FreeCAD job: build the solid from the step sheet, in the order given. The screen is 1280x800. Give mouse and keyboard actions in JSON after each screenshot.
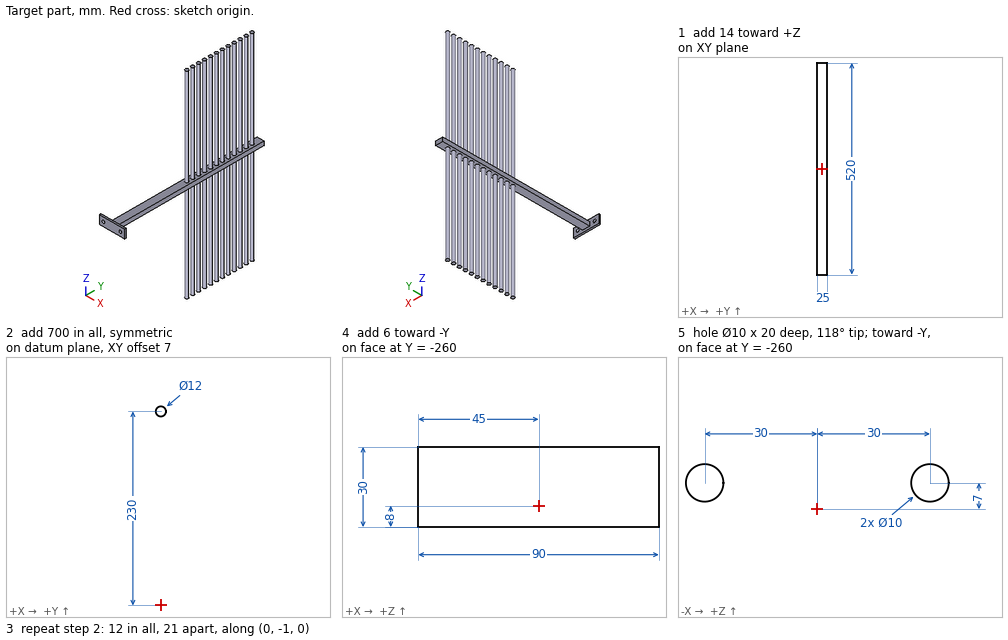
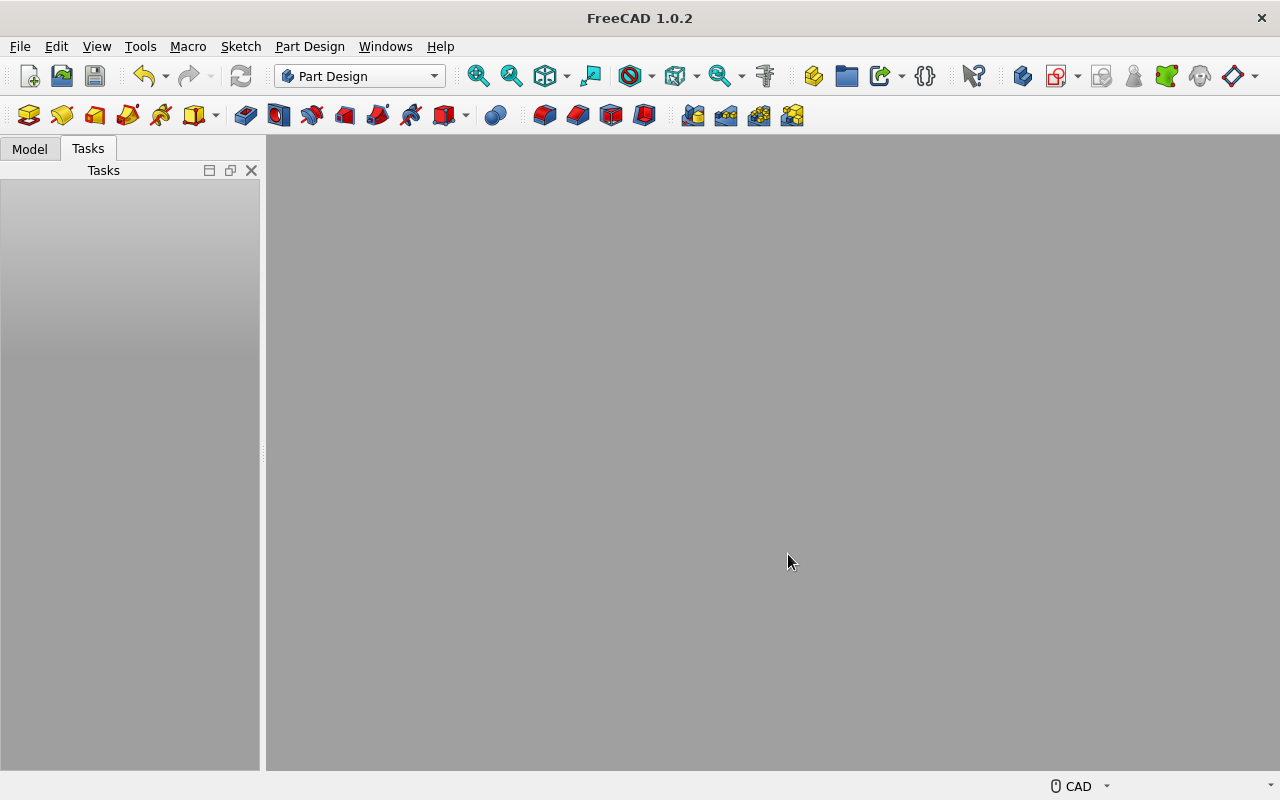
{"action": "left_click", "coordinate": [29, 76]}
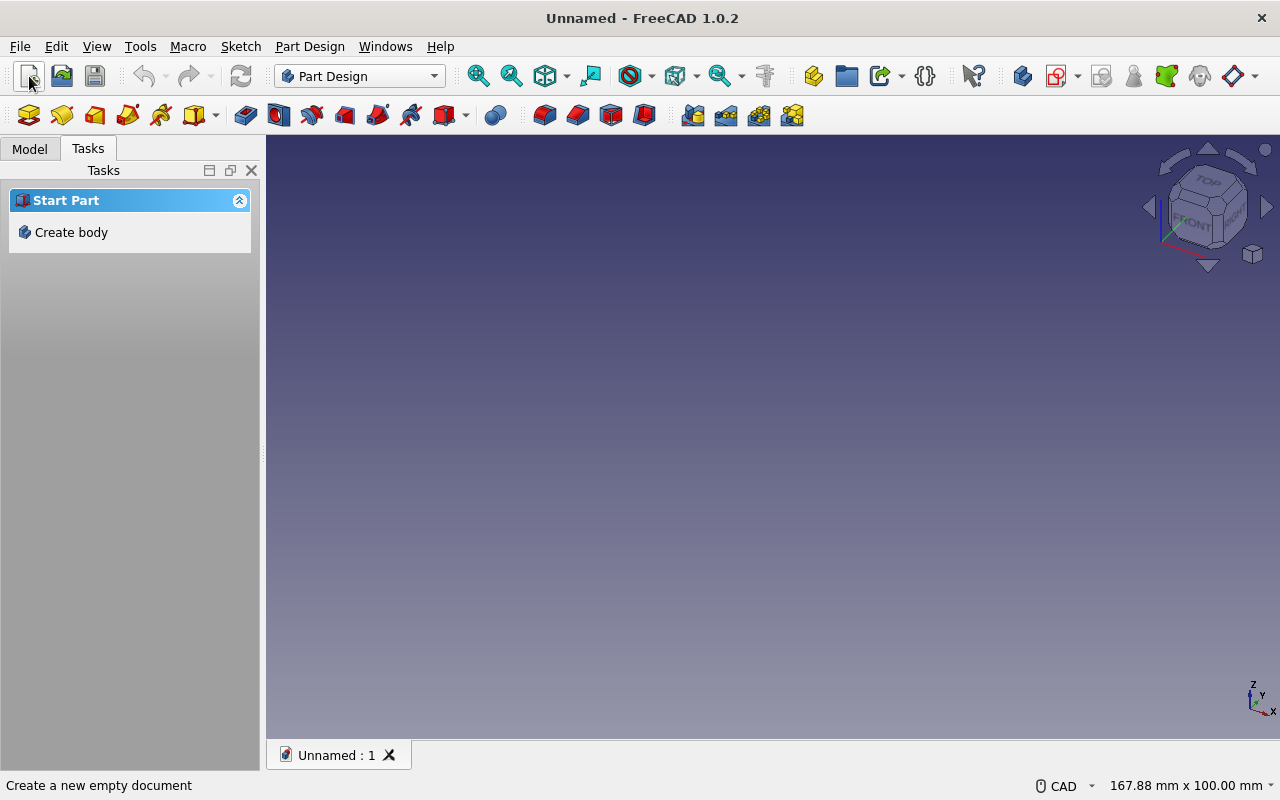
{"action": "left_click", "coordinate": [1056, 76]}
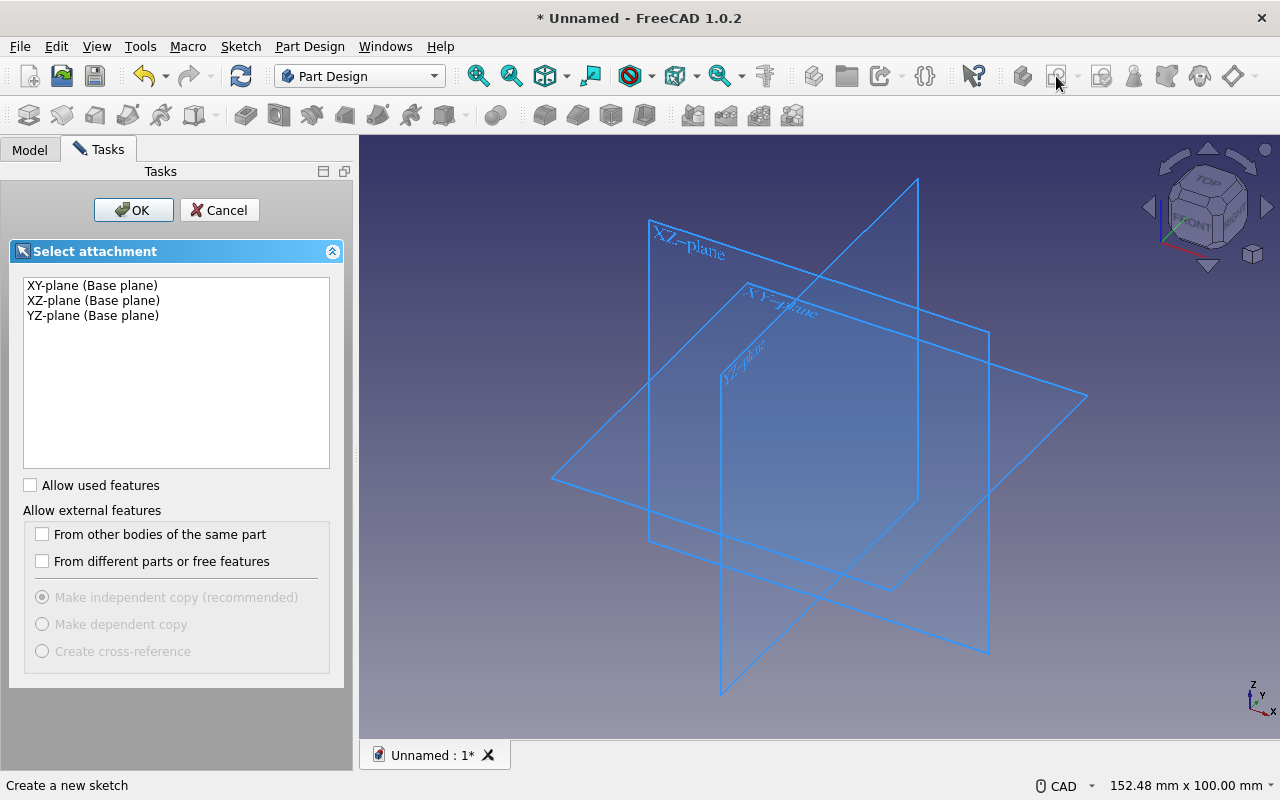
{"action": "left_click", "coordinate": [84, 286]}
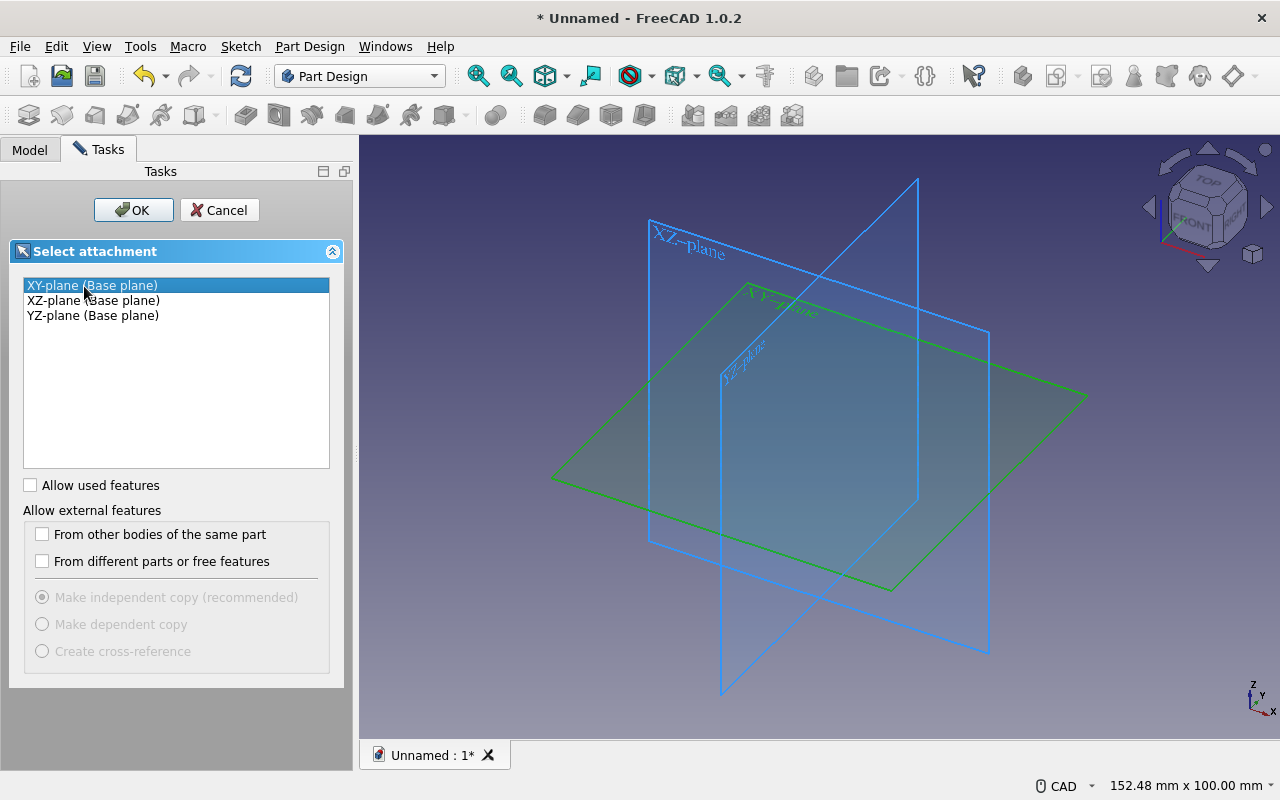
{"action": "left_click", "coordinate": [134, 210]}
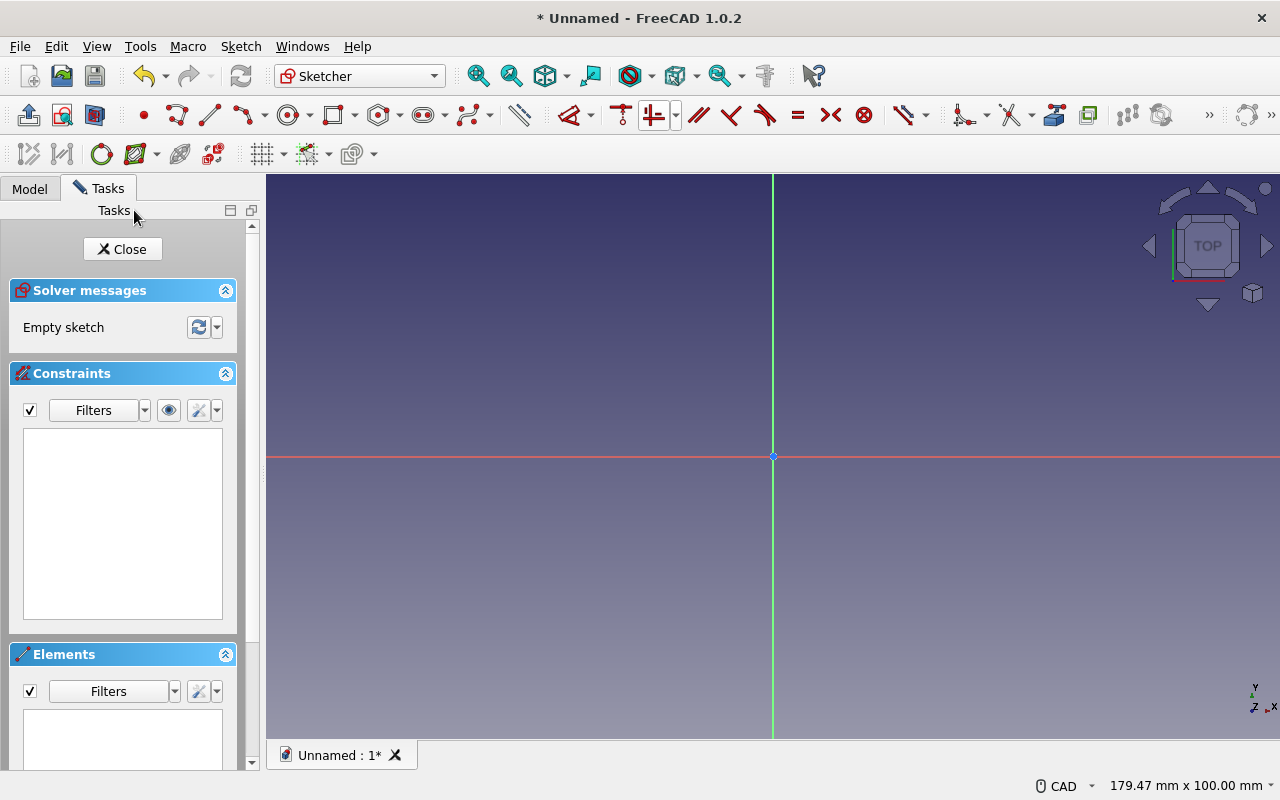
{"action": "scroll", "coordinate": [696, 456], "scroll_direction": "down", "scroll_amount": 11}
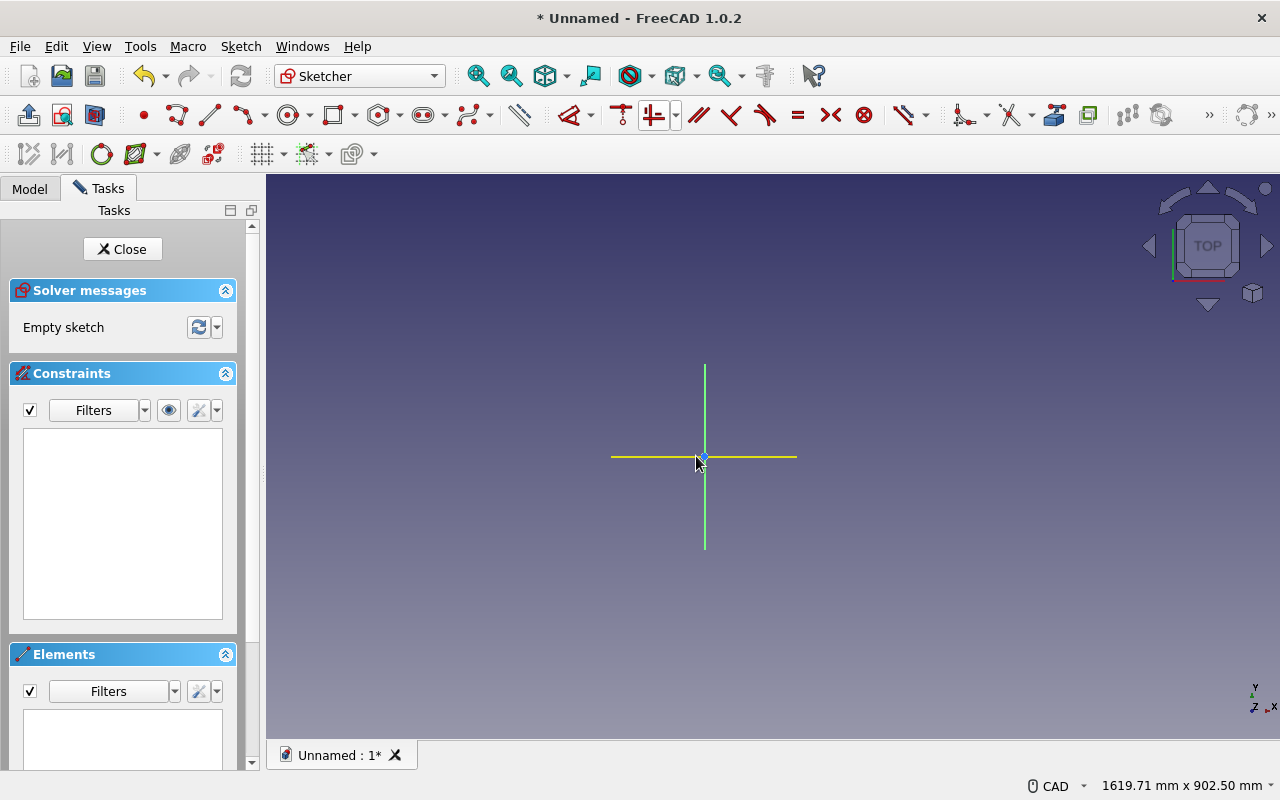
{"action": "left_click", "coordinate": [354, 116]}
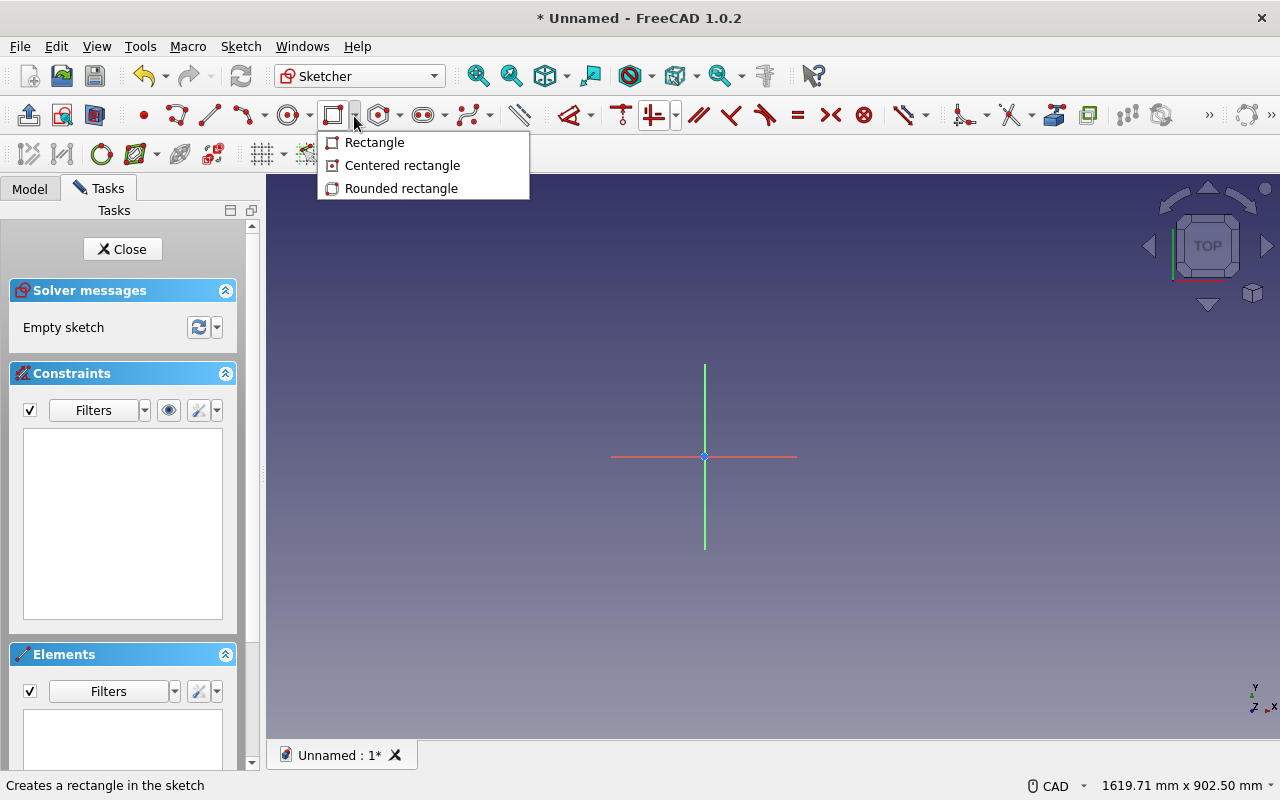
{"action": "left_click", "coordinate": [424, 166]}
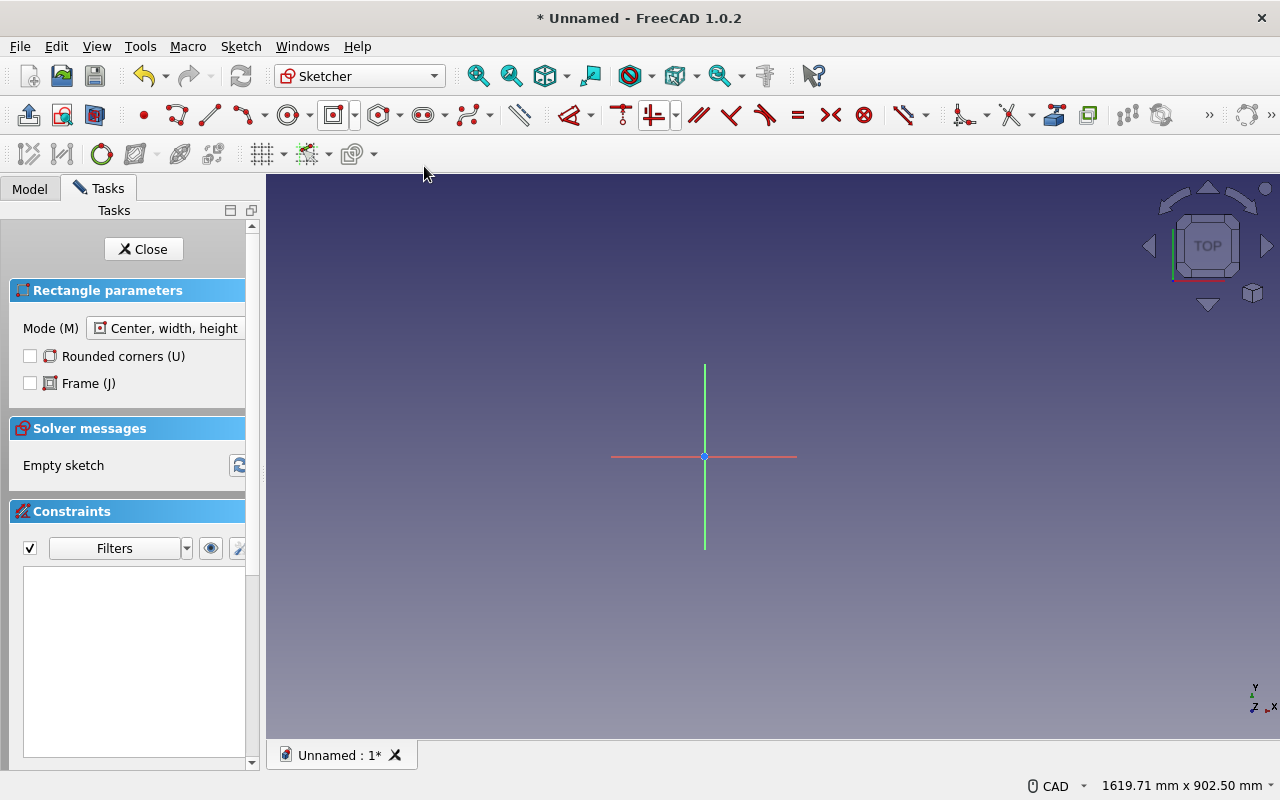
{"action": "scroll", "coordinate": [705, 456], "scroll_direction": "up", "scroll_amount": 4}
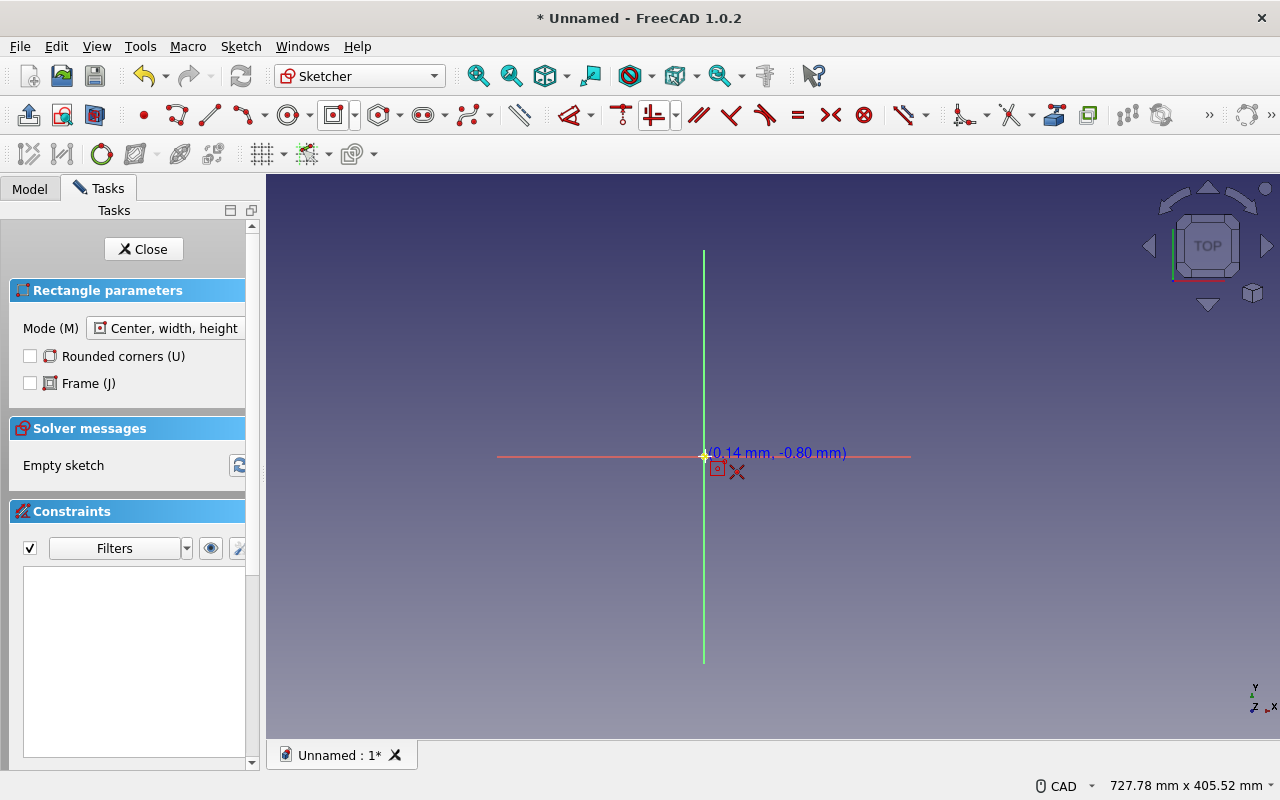
{"action": "left_click", "coordinate": [704, 456]}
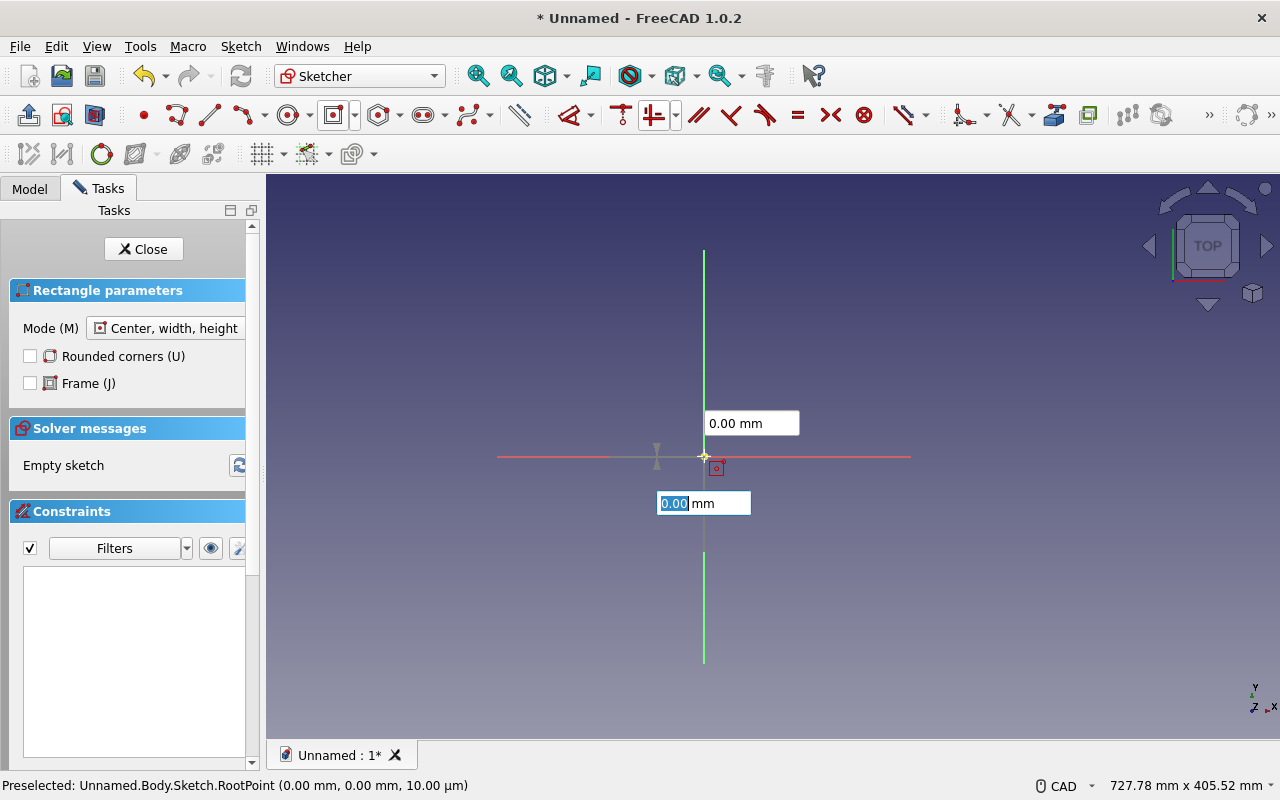
{"action": "scroll", "coordinate": [705, 456], "scroll_direction": "down", "scroll_amount": 4}